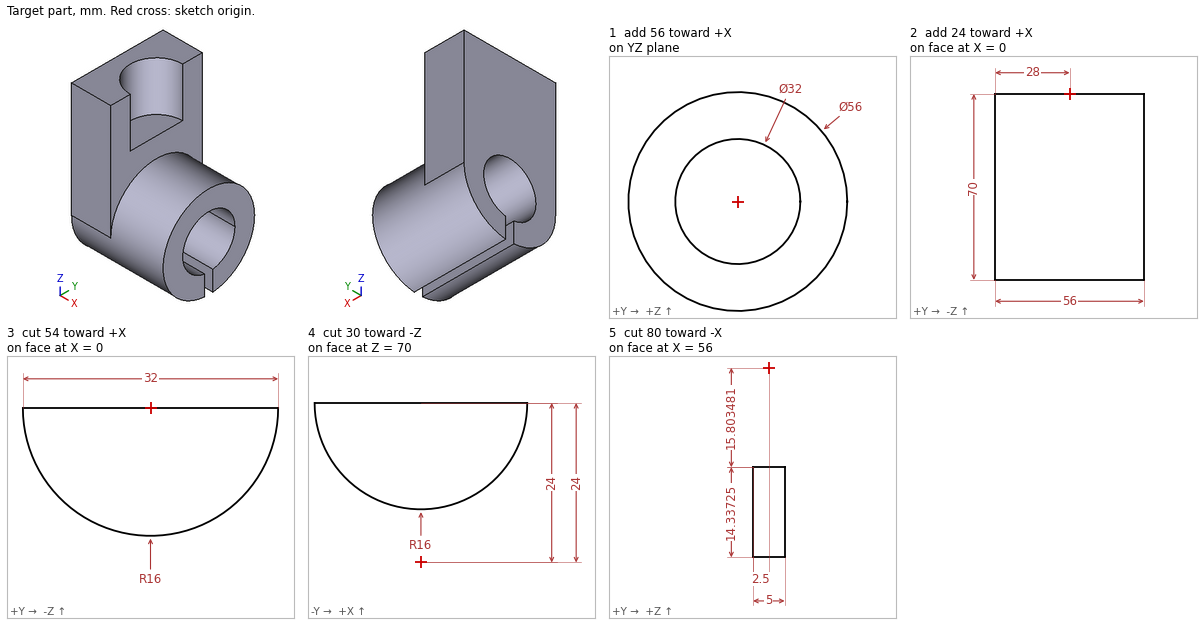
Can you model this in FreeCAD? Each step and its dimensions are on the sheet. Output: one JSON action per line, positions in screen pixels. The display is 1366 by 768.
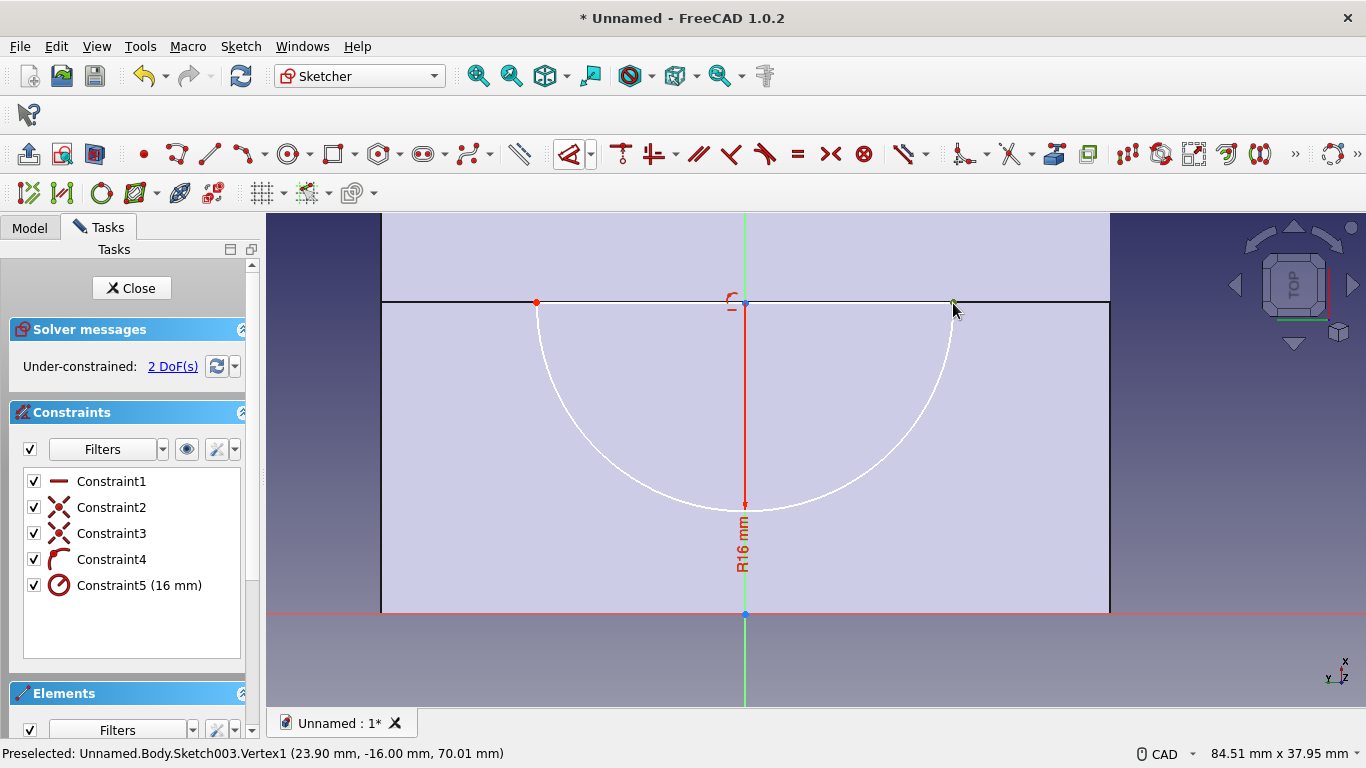
{"action": "left_click", "coordinate": [590, 154]}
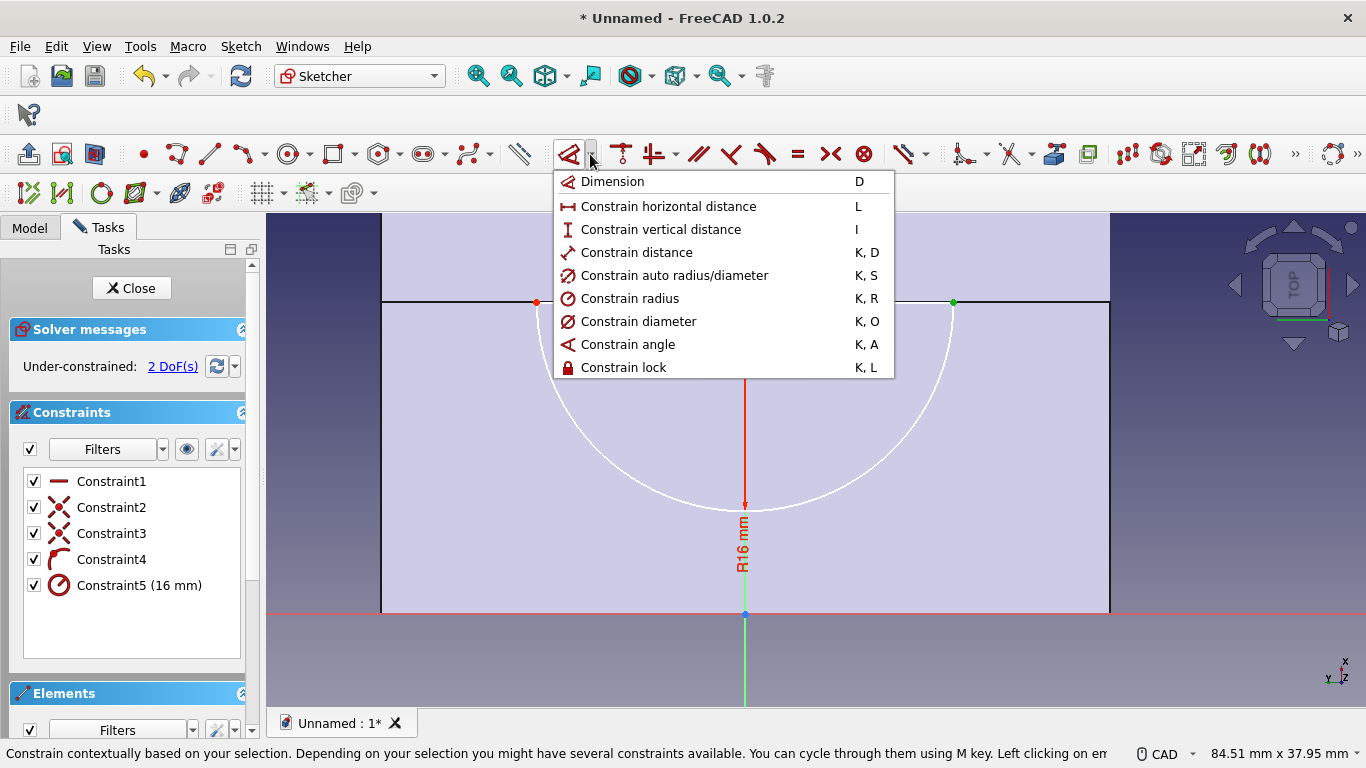
{"action": "left_click", "coordinate": [724, 230]}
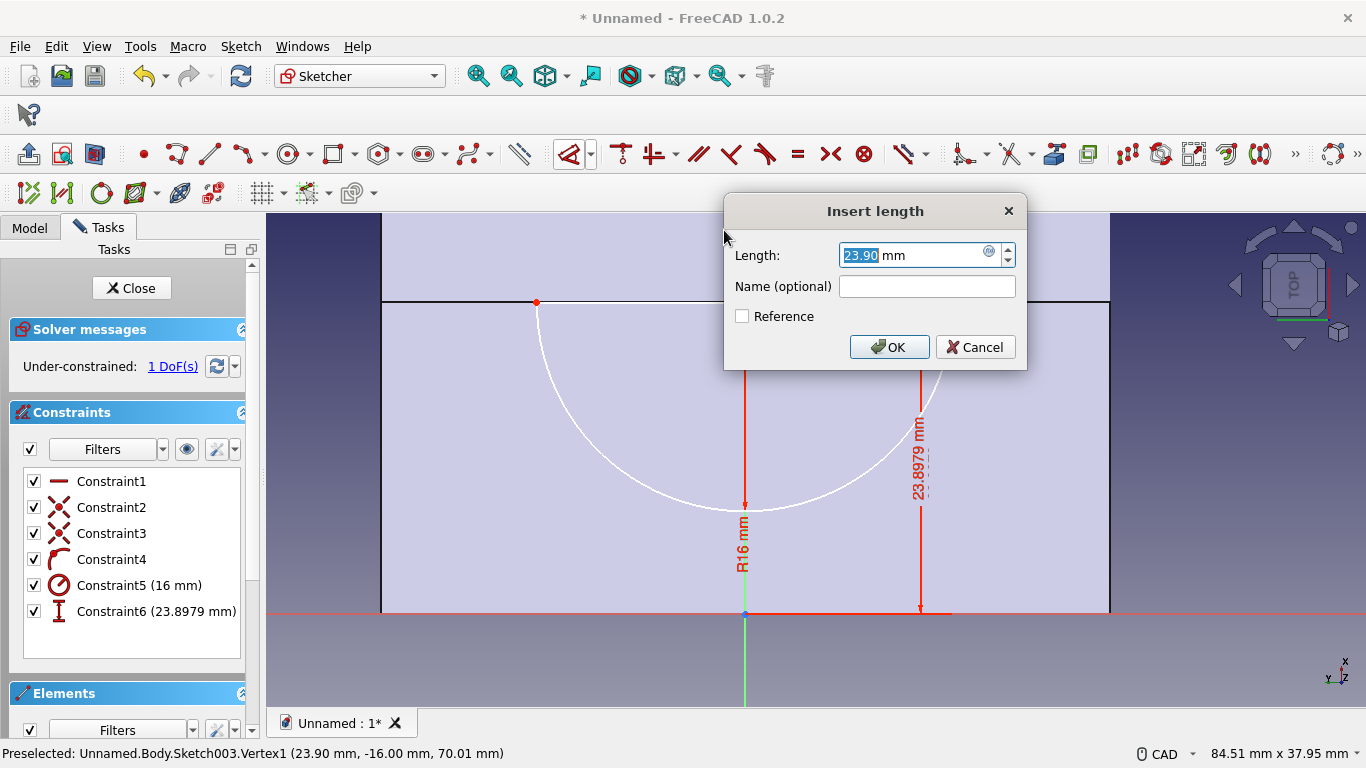
{"action": "type", "text": "24"}
{"action": "key", "text": "Return"}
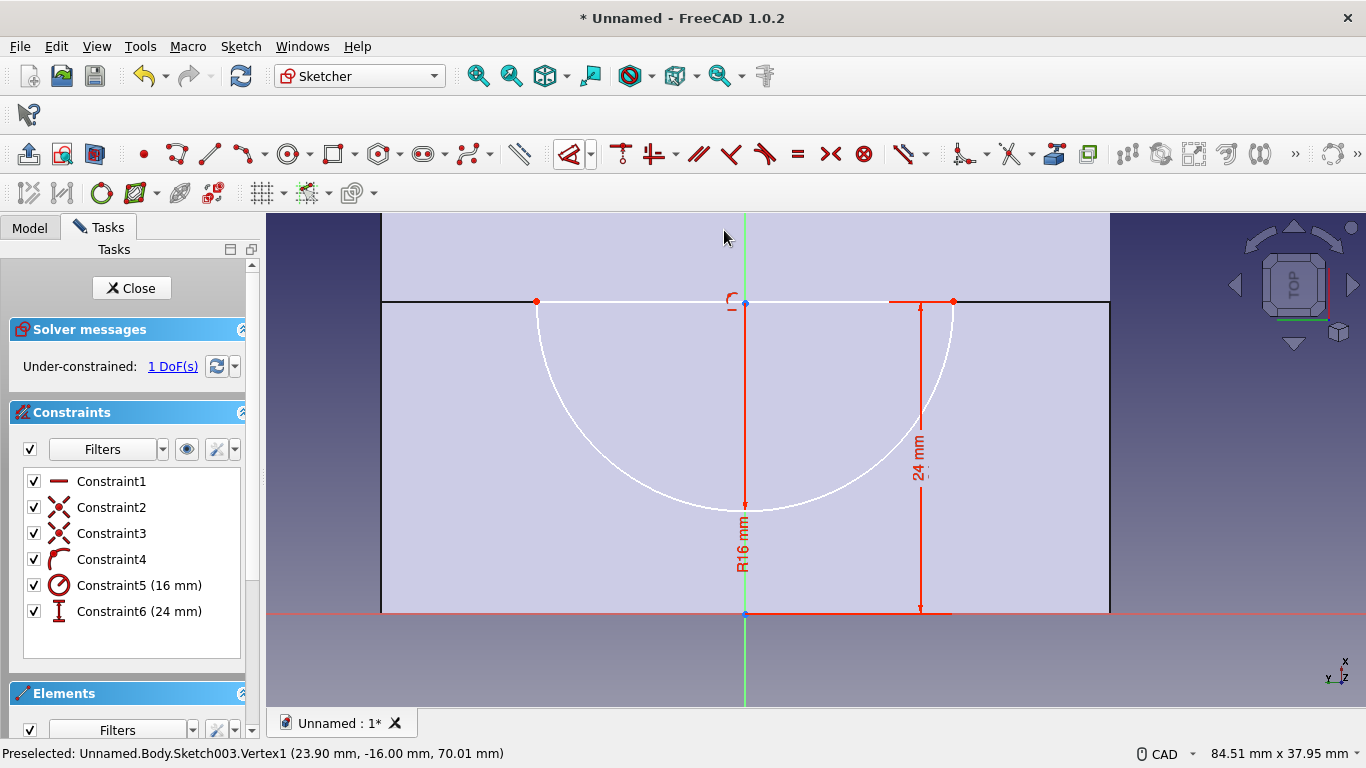
{"action": "left_click", "coordinate": [745, 303]}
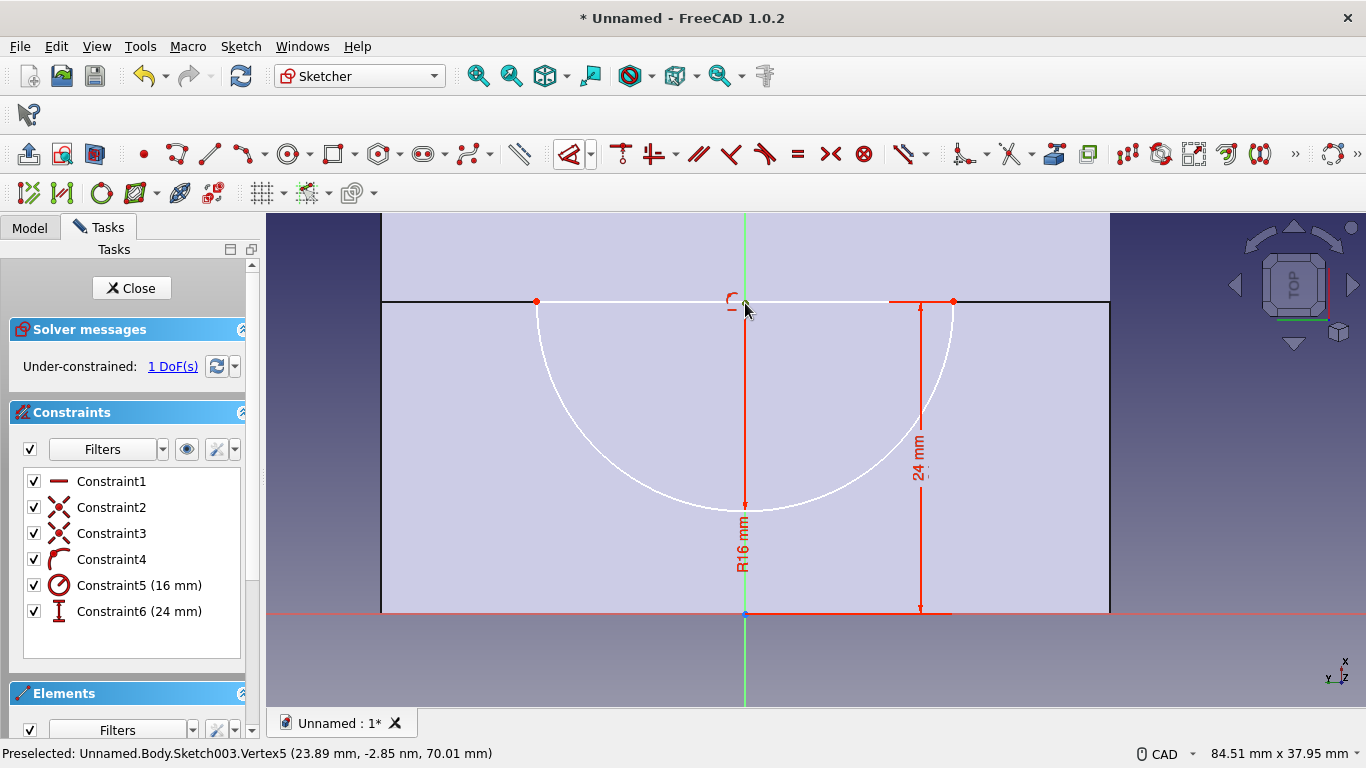
{"action": "key", "text": "i"}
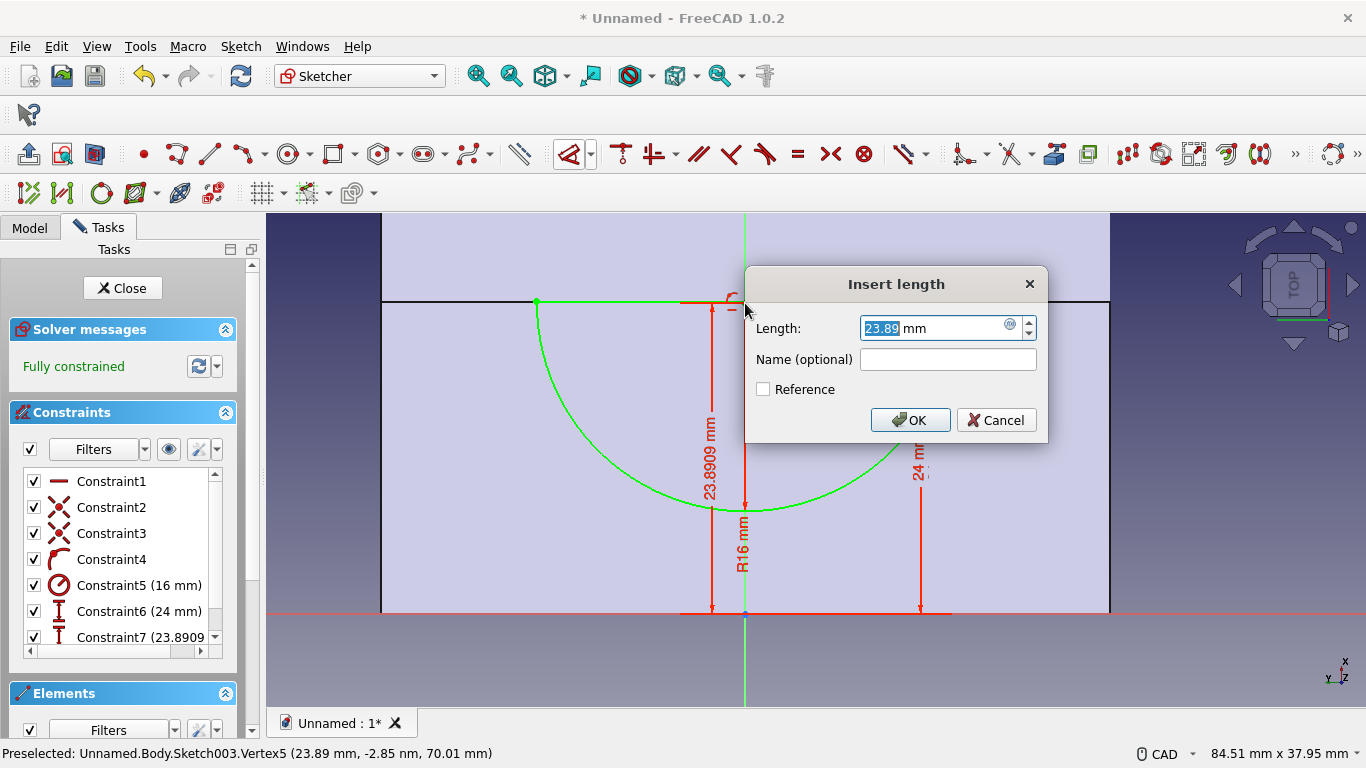
{"action": "type", "text": "24"}
{"action": "key", "text": "Return"}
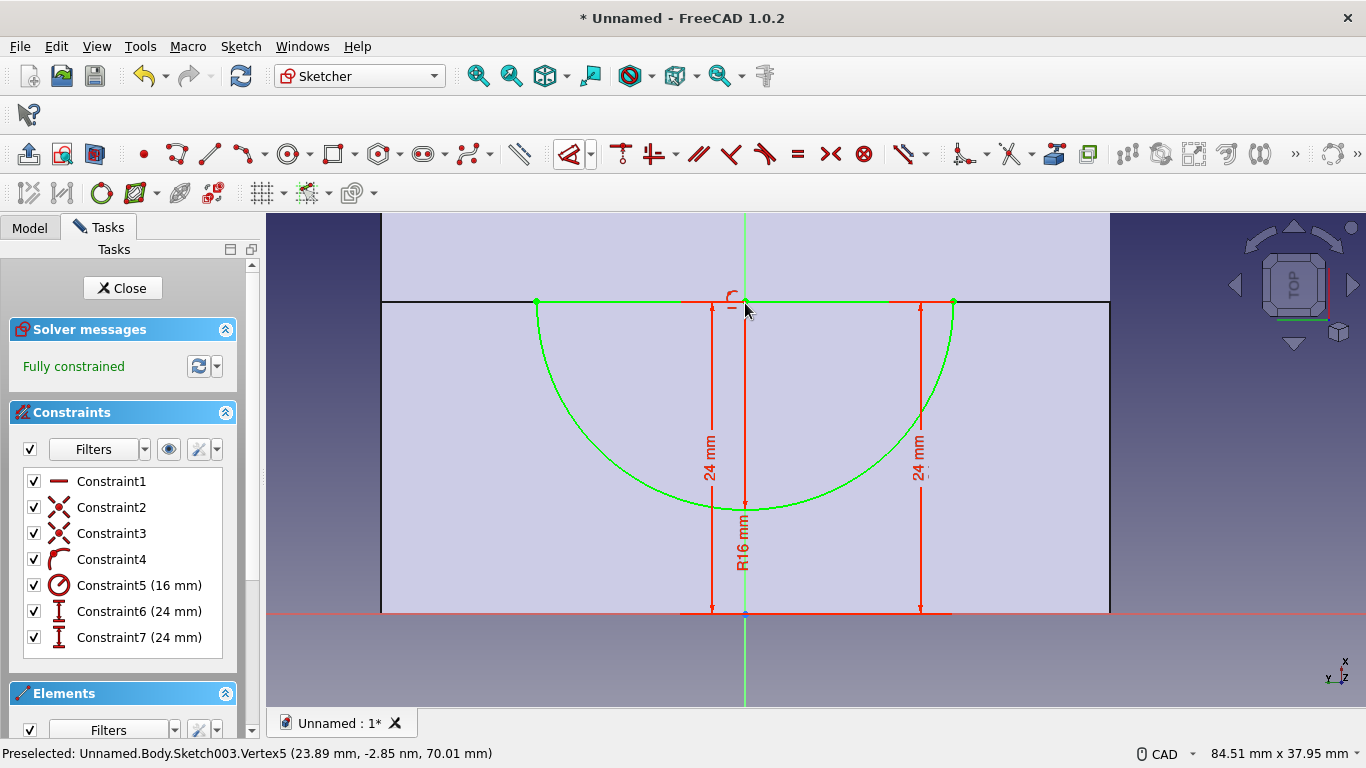
{"action": "left_click", "coordinate": [123, 288]}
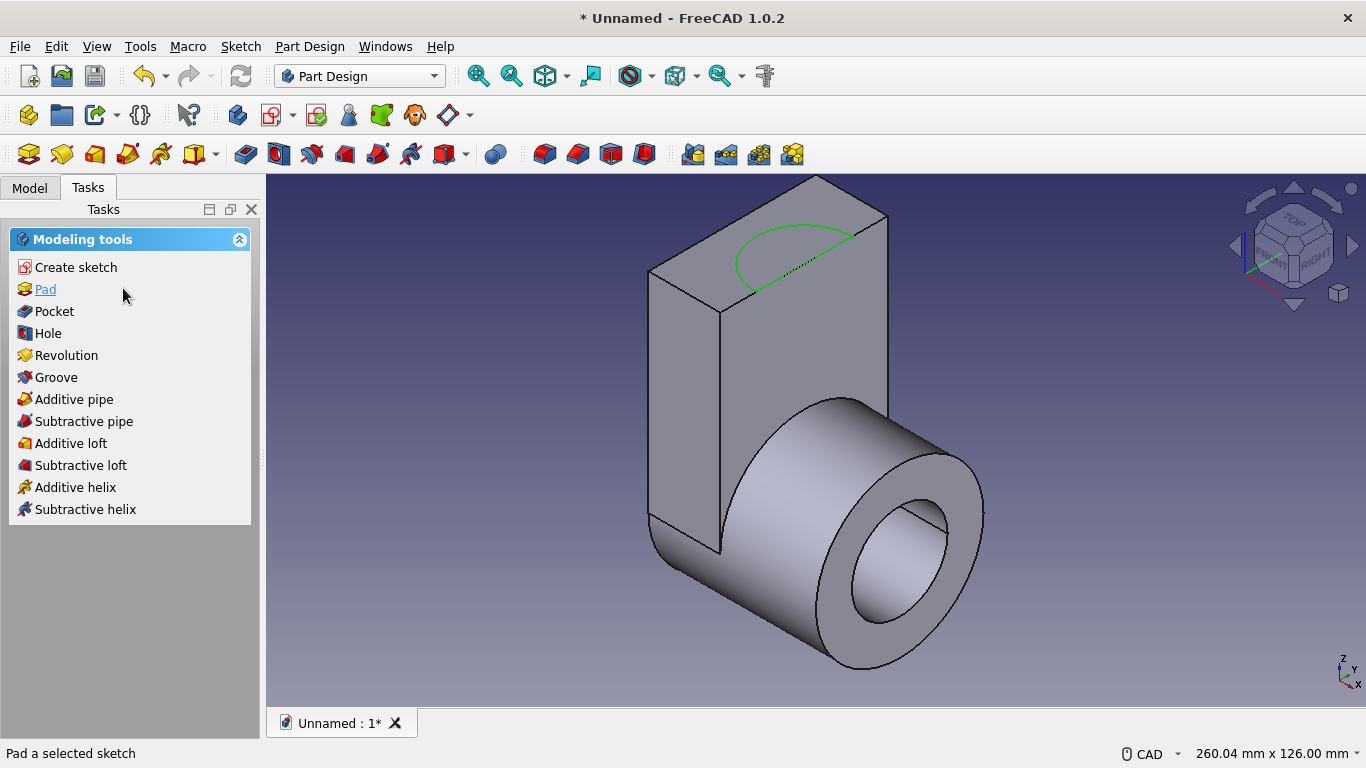
{"action": "left_click", "coordinate": [246, 154]}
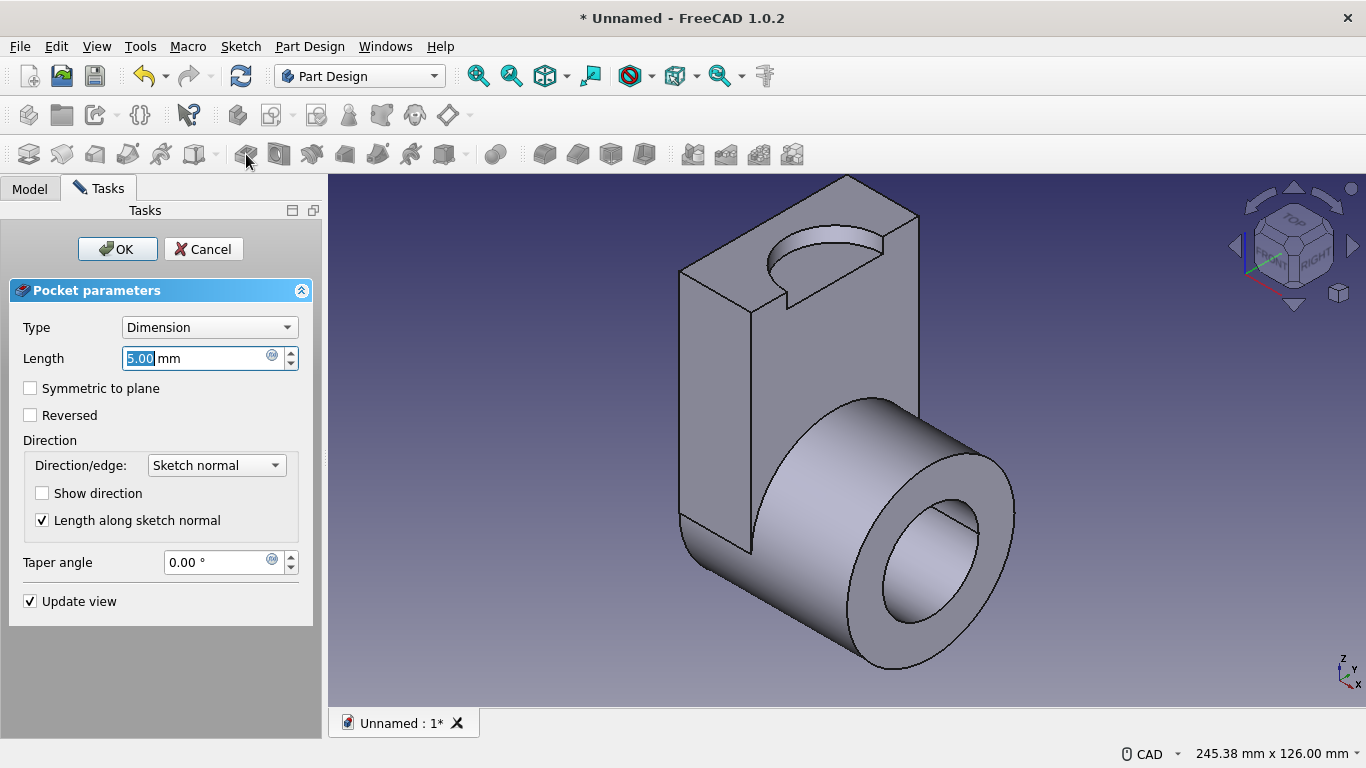
{"action": "type", "text": "30"}
{"action": "key", "text": "Tab"}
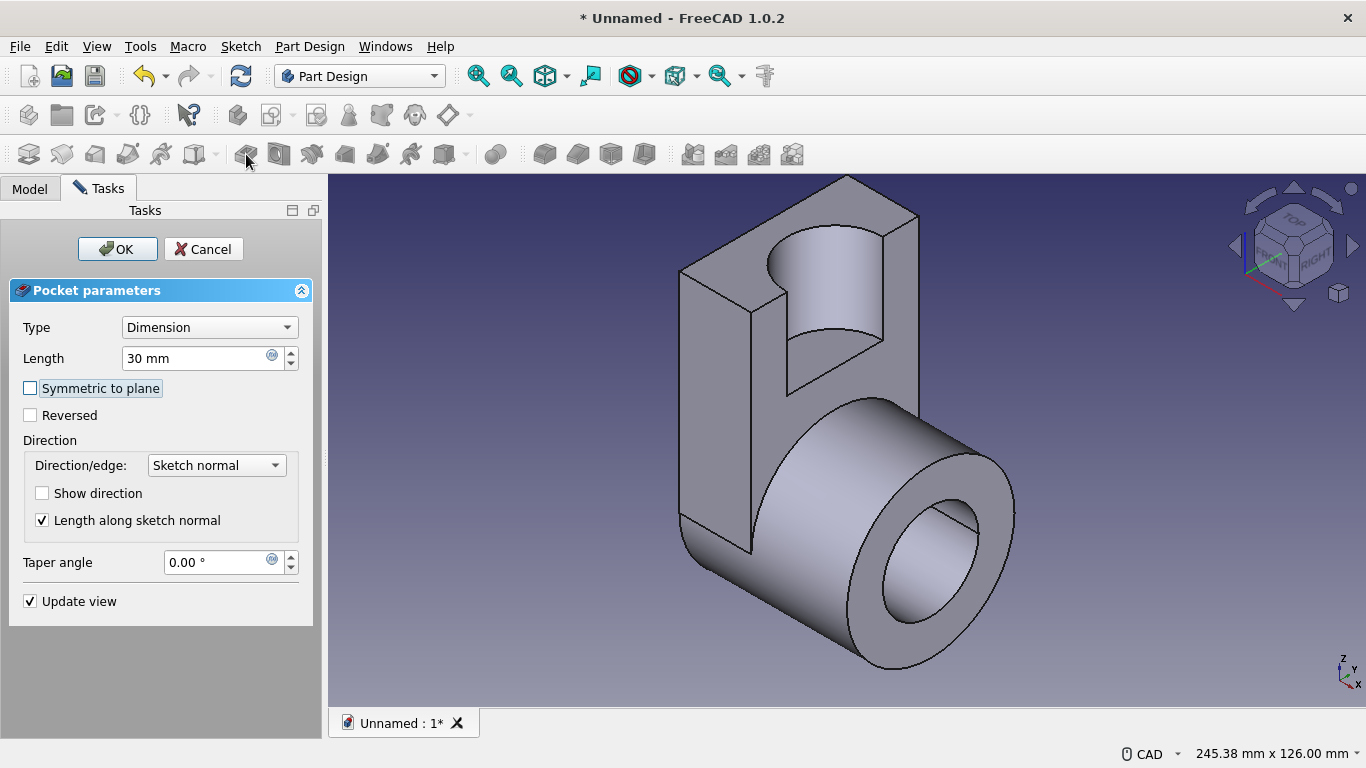
{"action": "left_click", "coordinate": [118, 249]}